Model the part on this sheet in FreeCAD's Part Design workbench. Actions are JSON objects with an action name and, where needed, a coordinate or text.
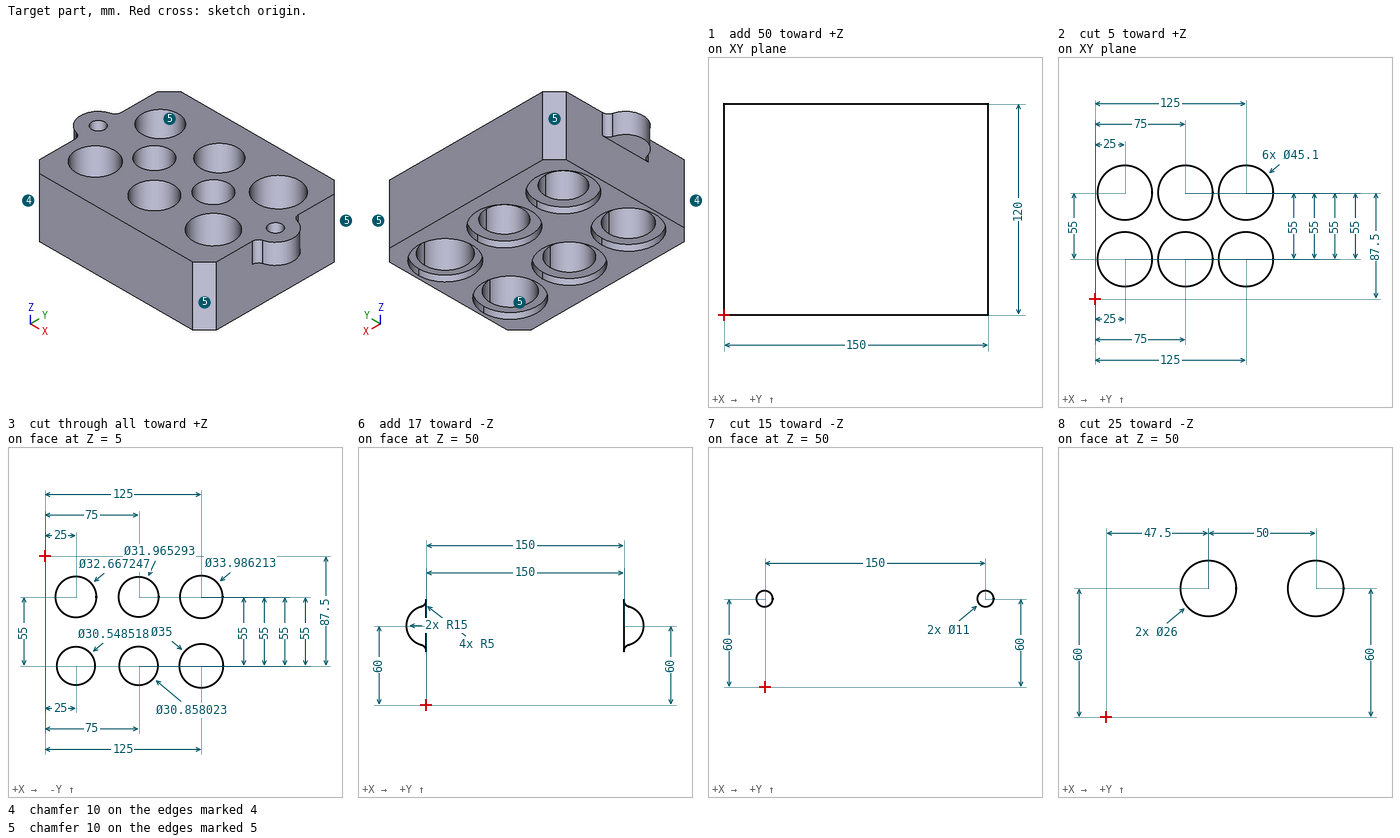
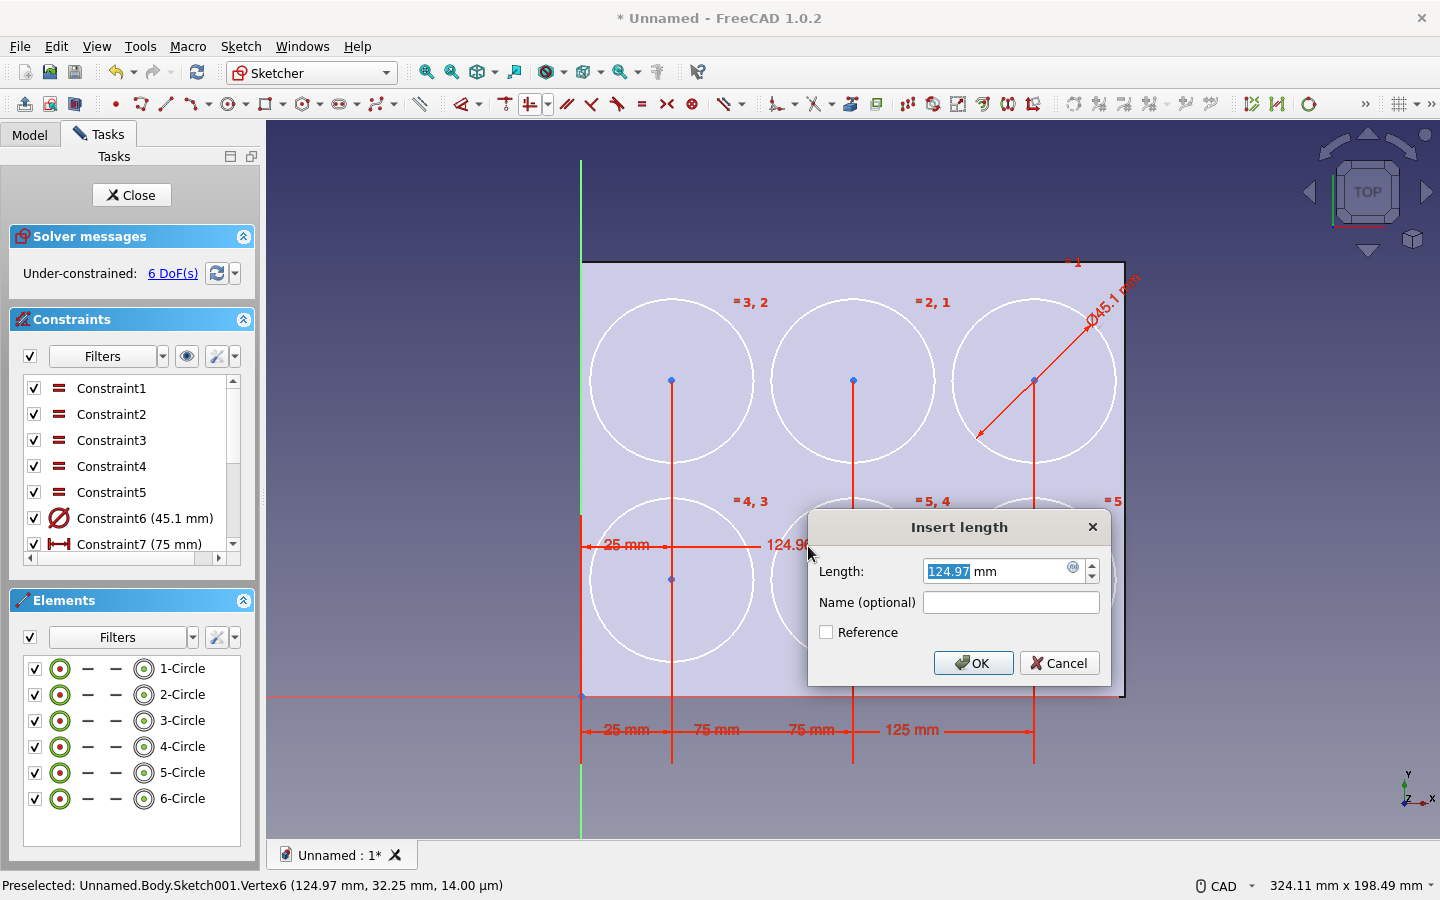
{"action": "type", "text": "125"}
{"action": "key", "text": "Return"}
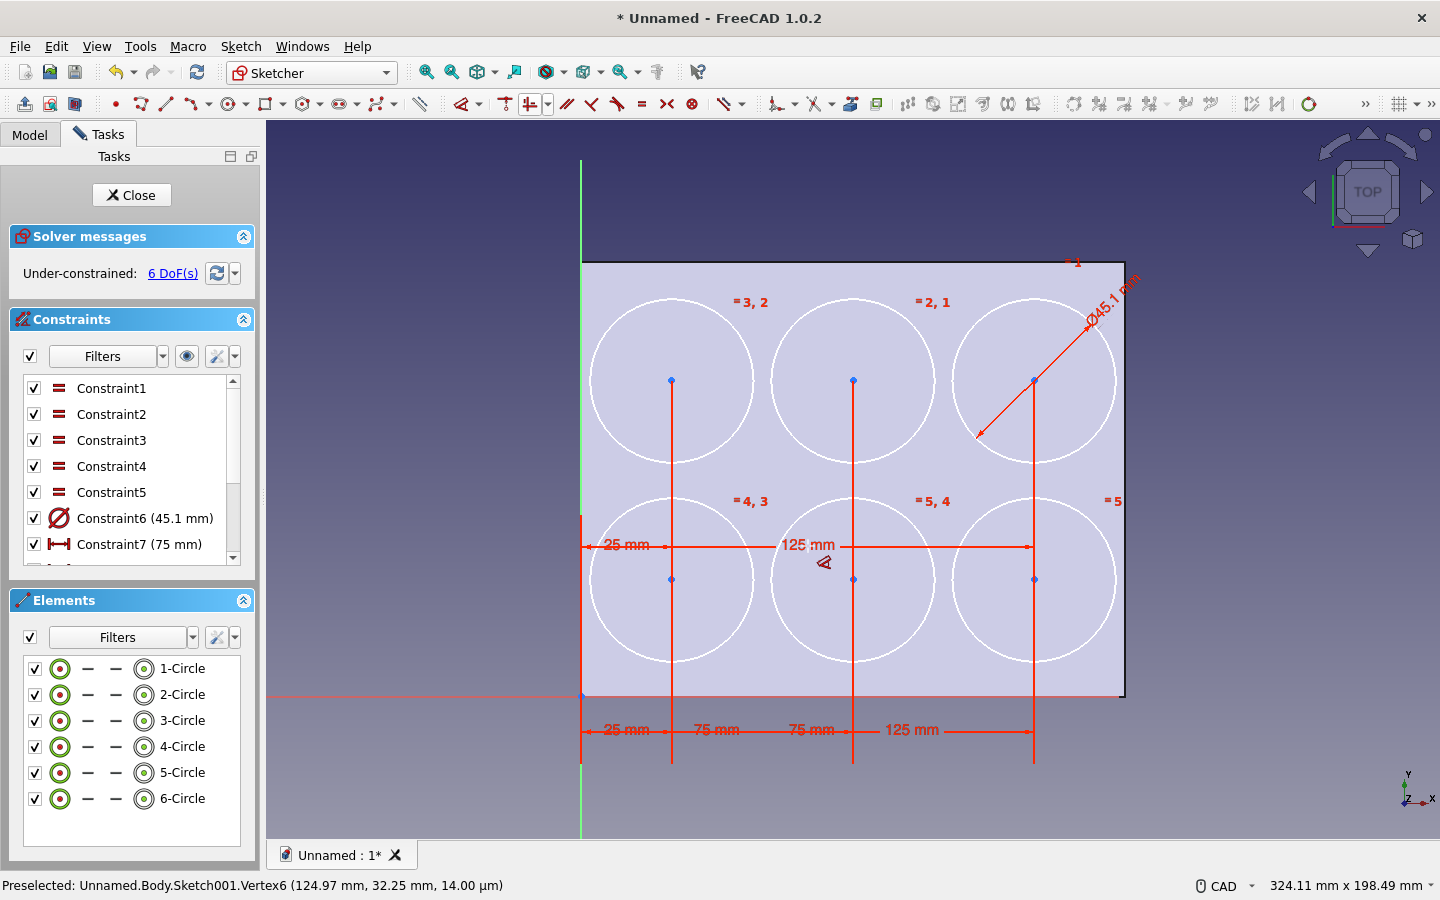
{"action": "left_click", "coordinate": [672, 381]}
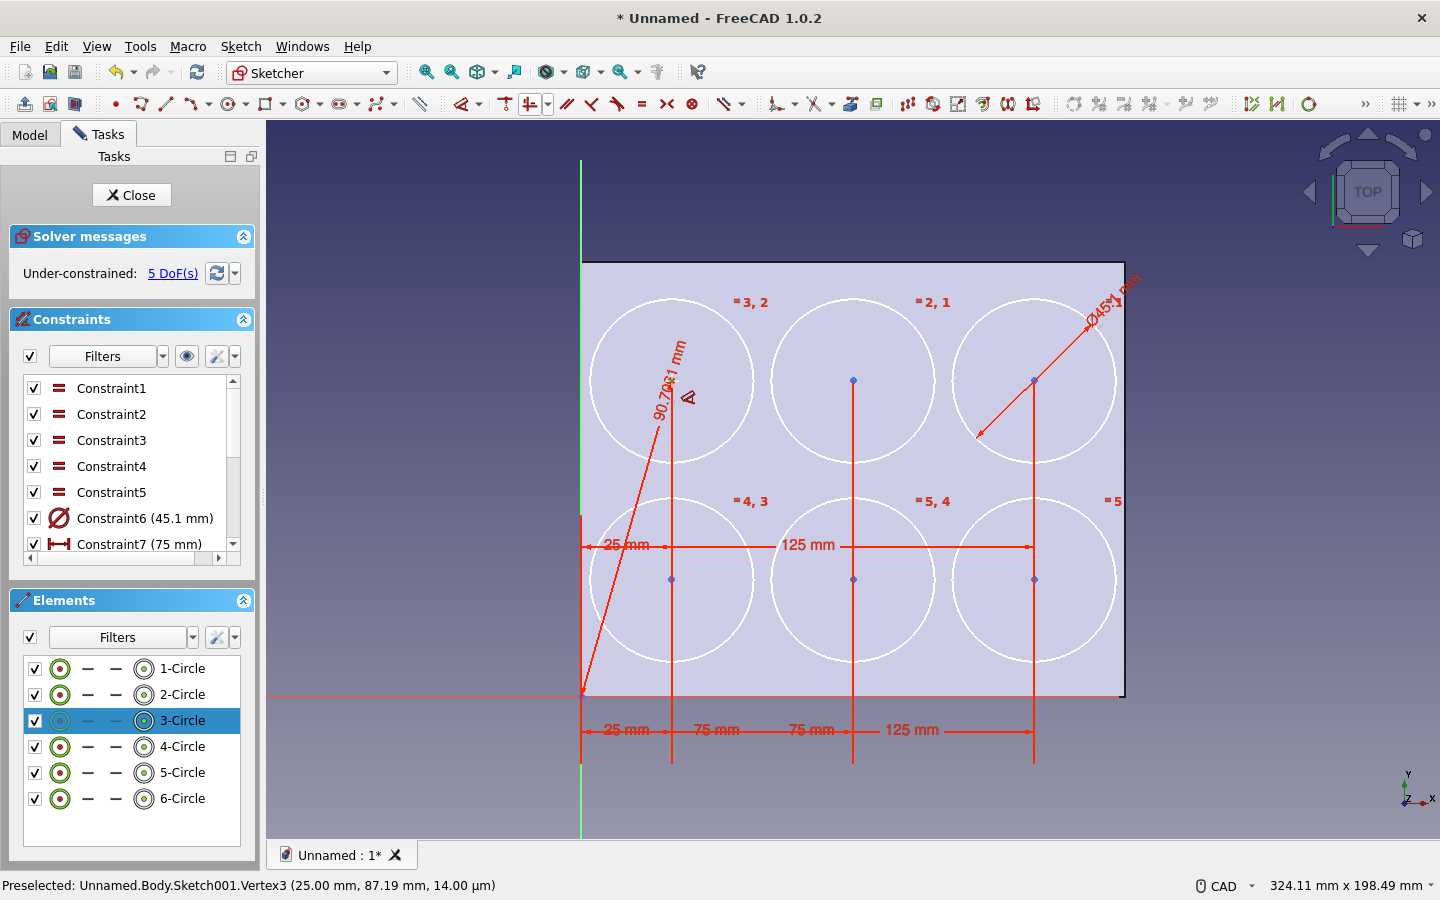
{"action": "left_click", "coordinate": [672, 580]}
{"action": "left_click", "coordinate": [638, 480]}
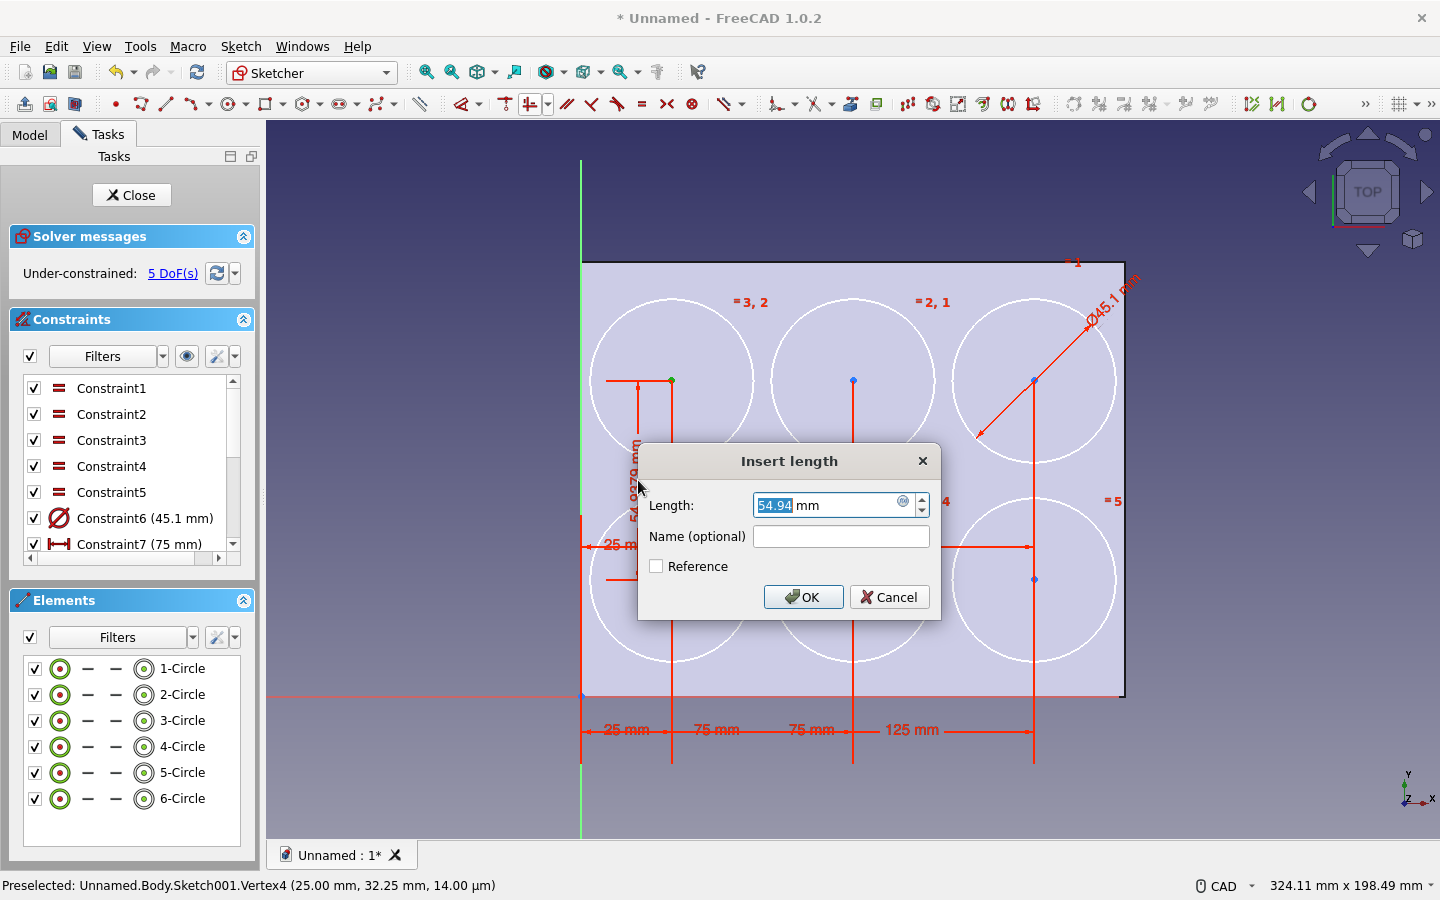
{"action": "type", "text": "55"}
{"action": "key", "text": "Return"}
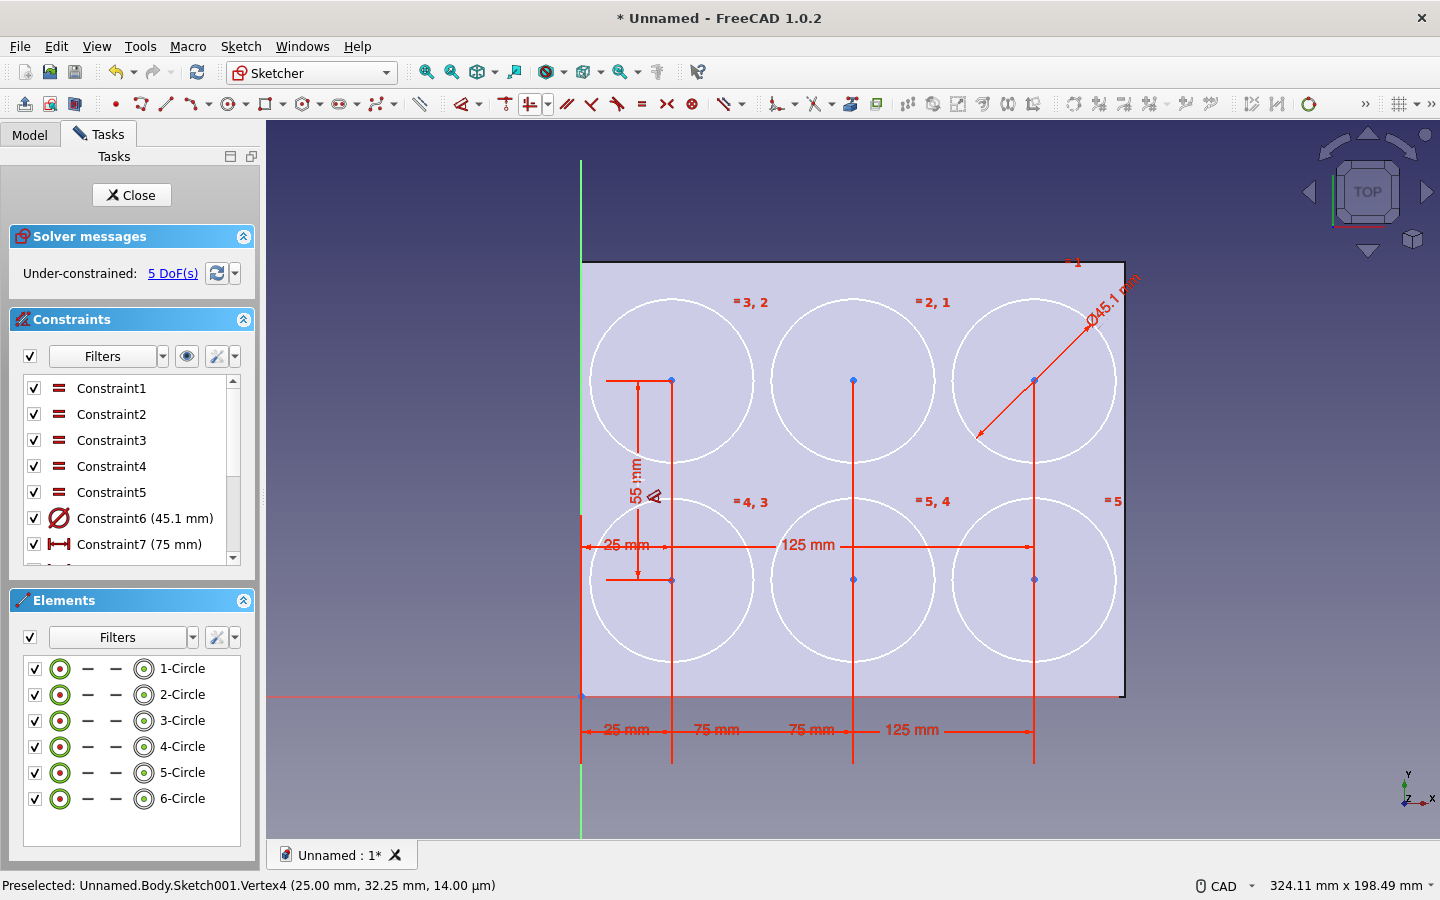
{"action": "left_click", "coordinate": [853, 381]}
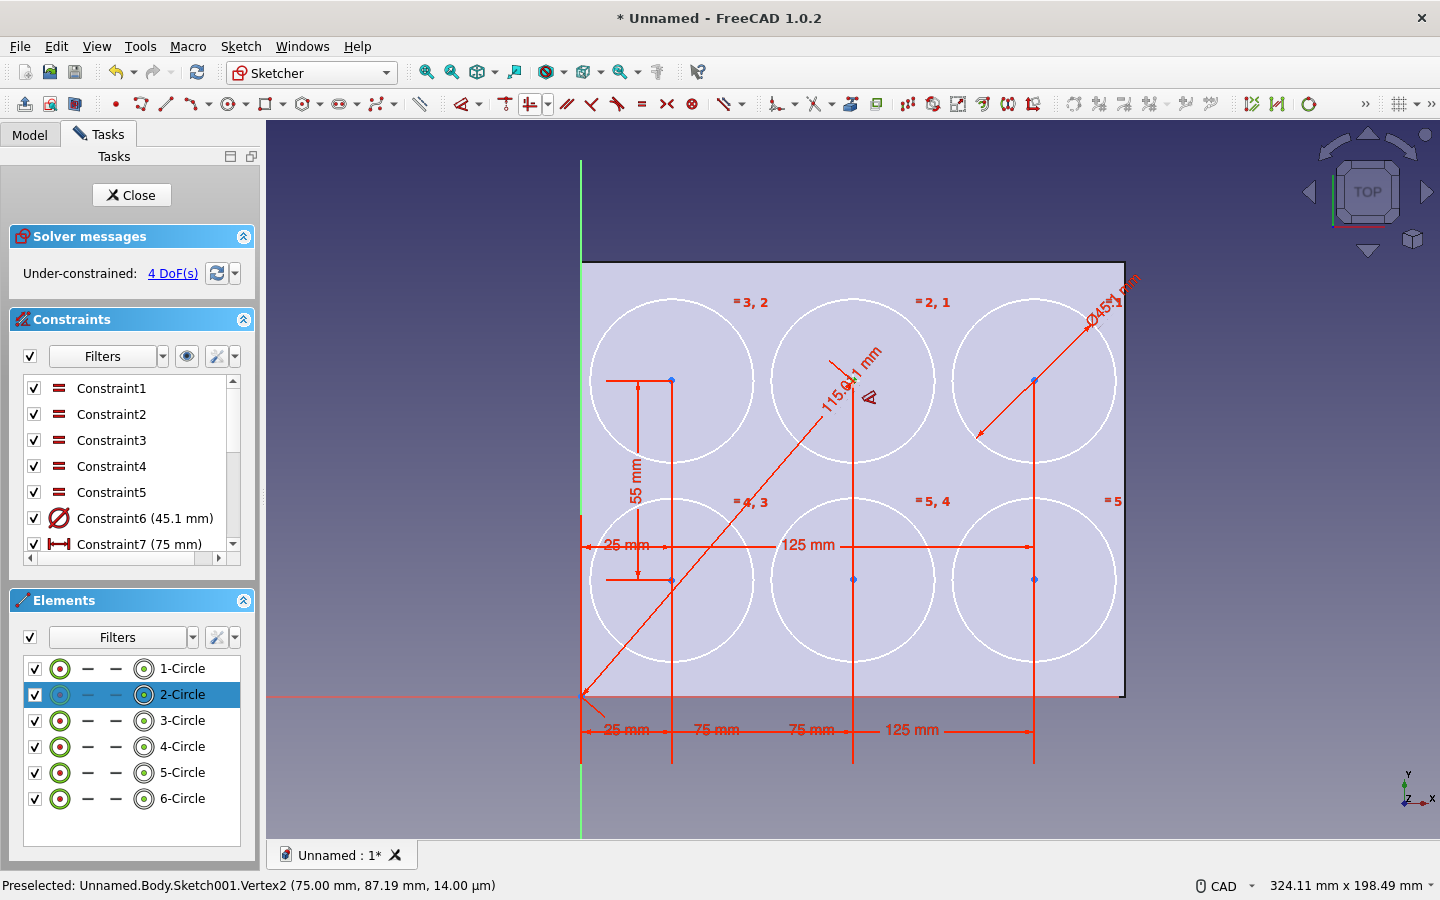
{"action": "left_click", "coordinate": [672, 580]}
{"action": "left_click", "coordinate": [638, 435]}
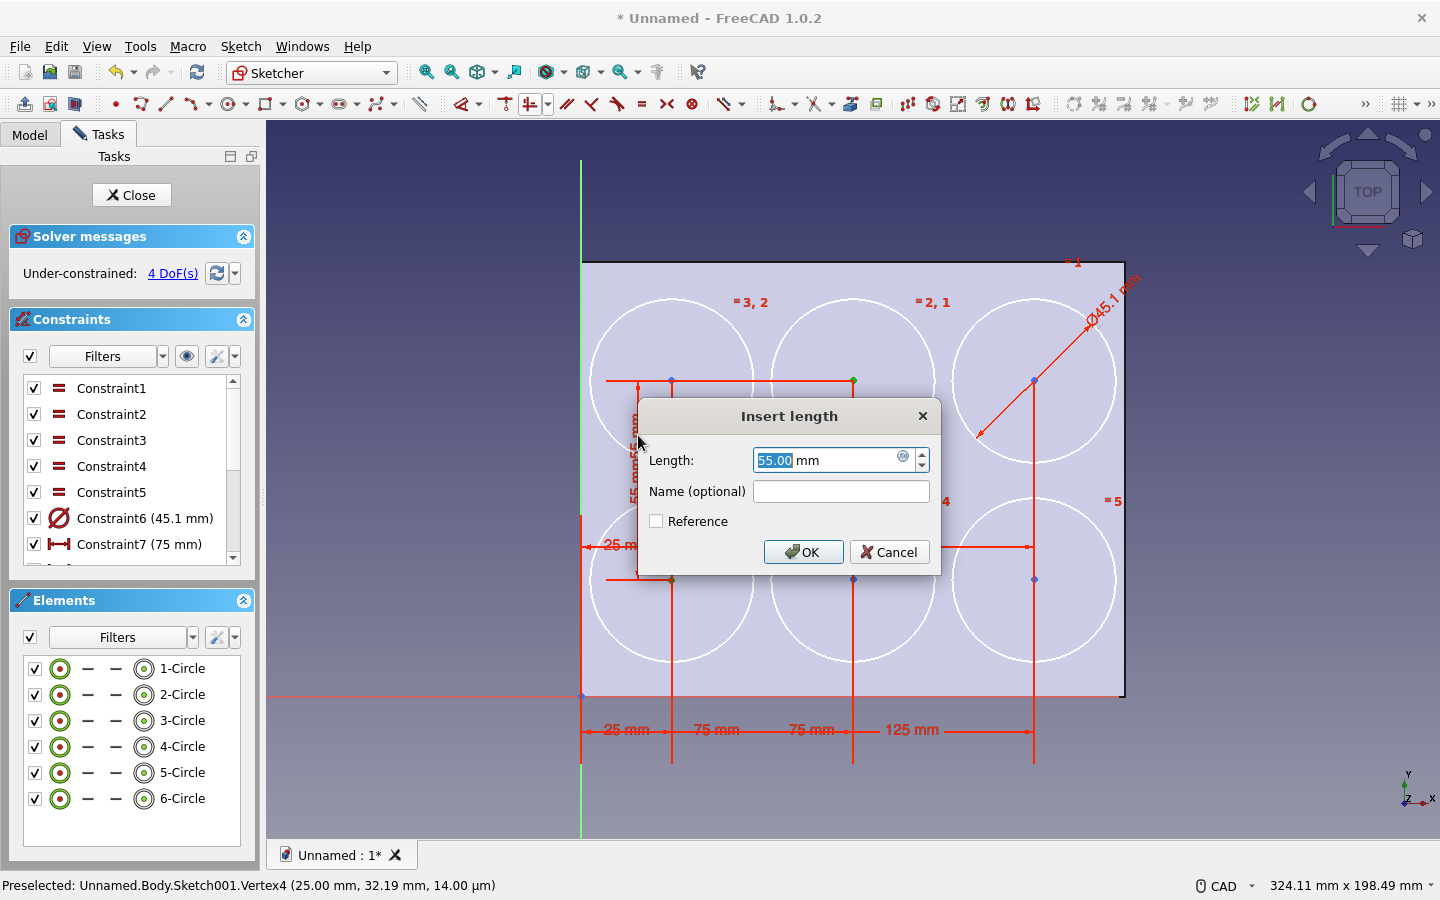
{"action": "type", "text": "55"}
{"action": "key", "text": "Return"}